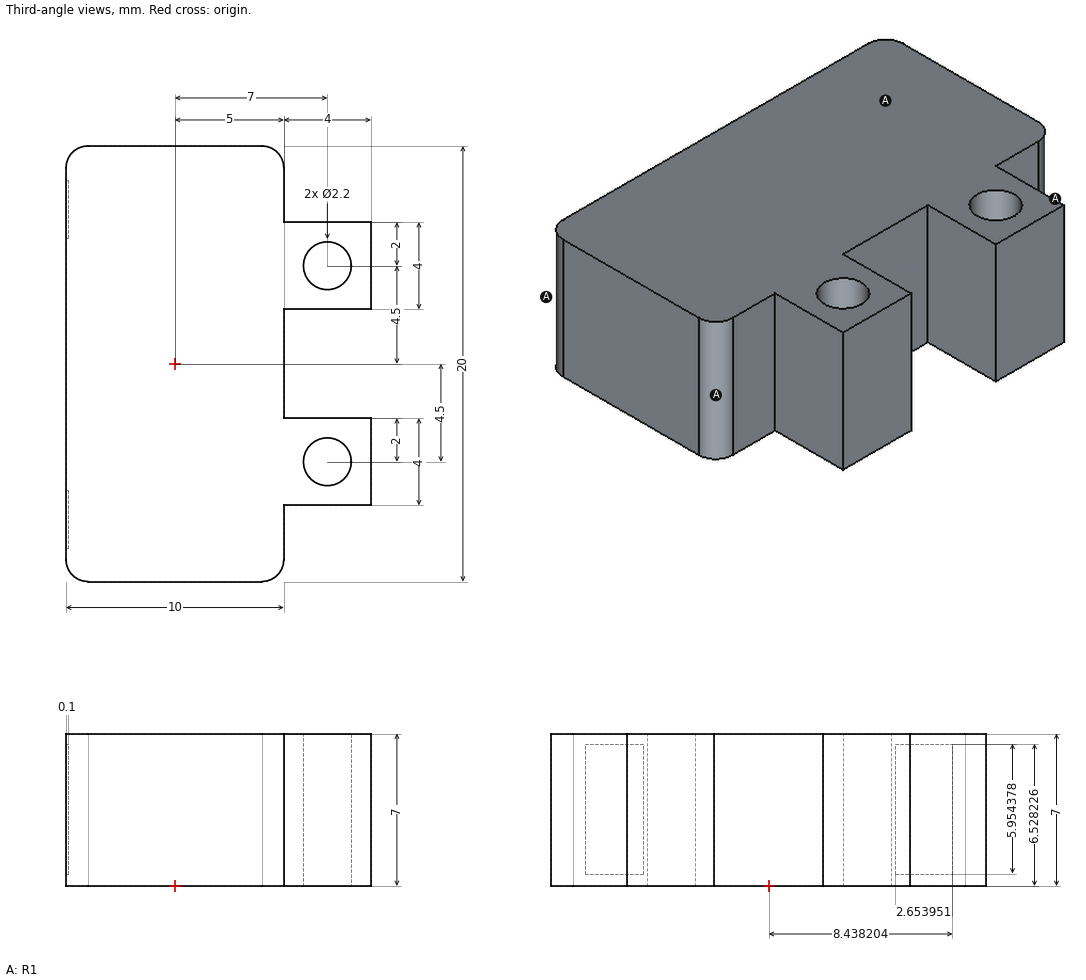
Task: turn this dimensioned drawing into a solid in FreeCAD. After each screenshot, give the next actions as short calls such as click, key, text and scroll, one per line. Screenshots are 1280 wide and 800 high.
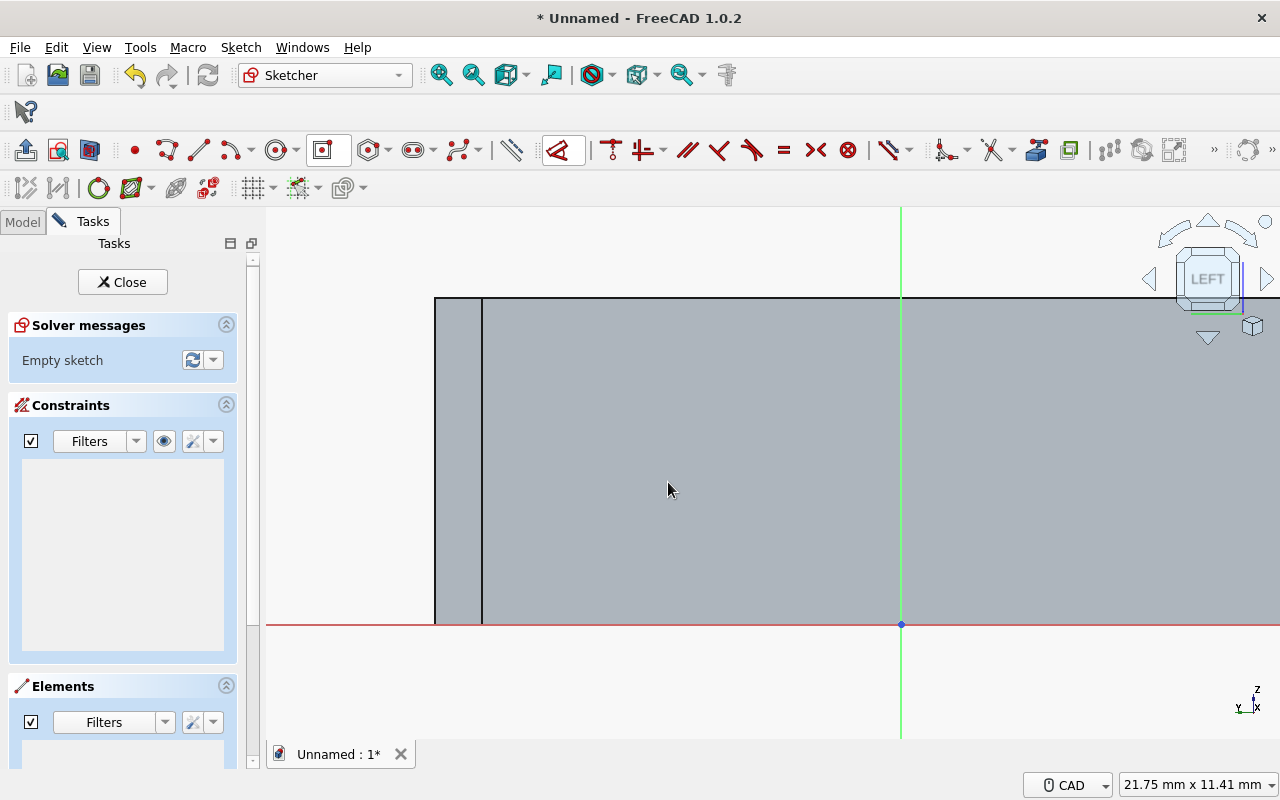
key(g)
key(r)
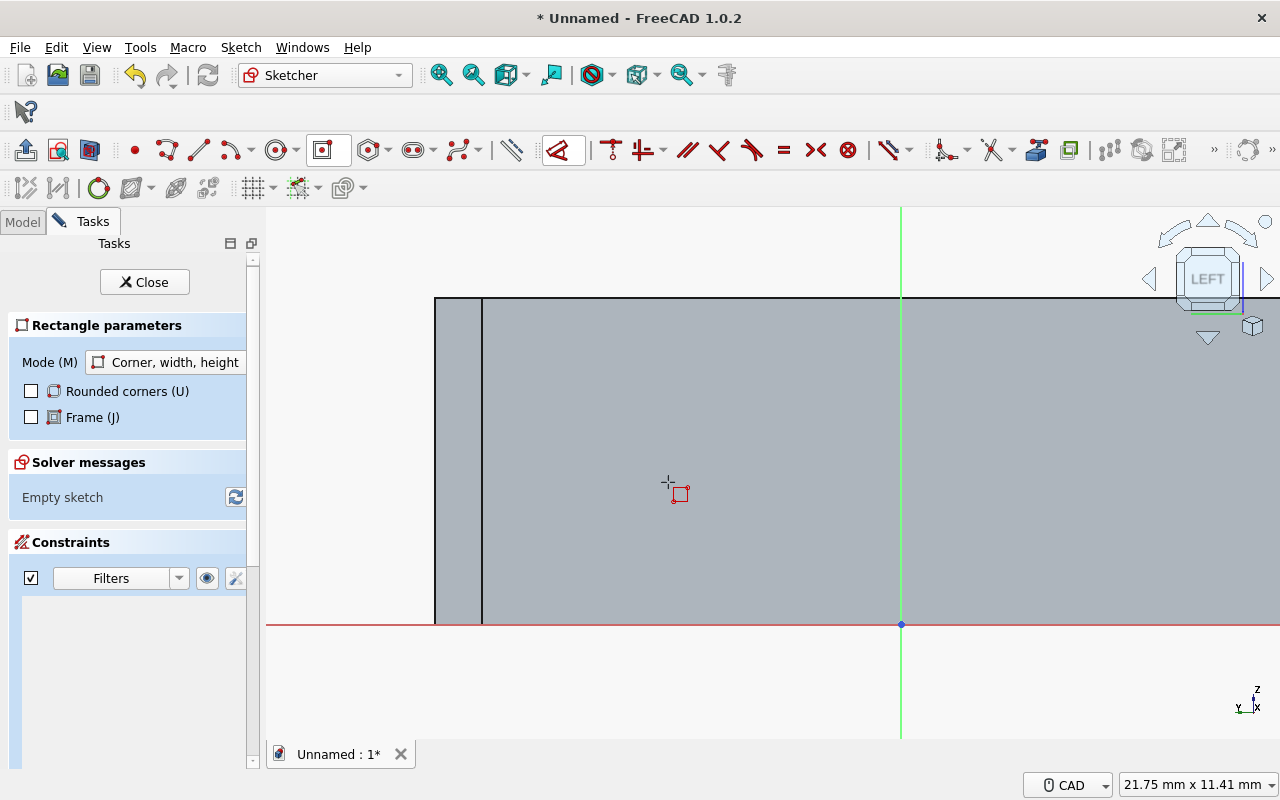
click(508, 320)
click(632, 598)
key(Escape)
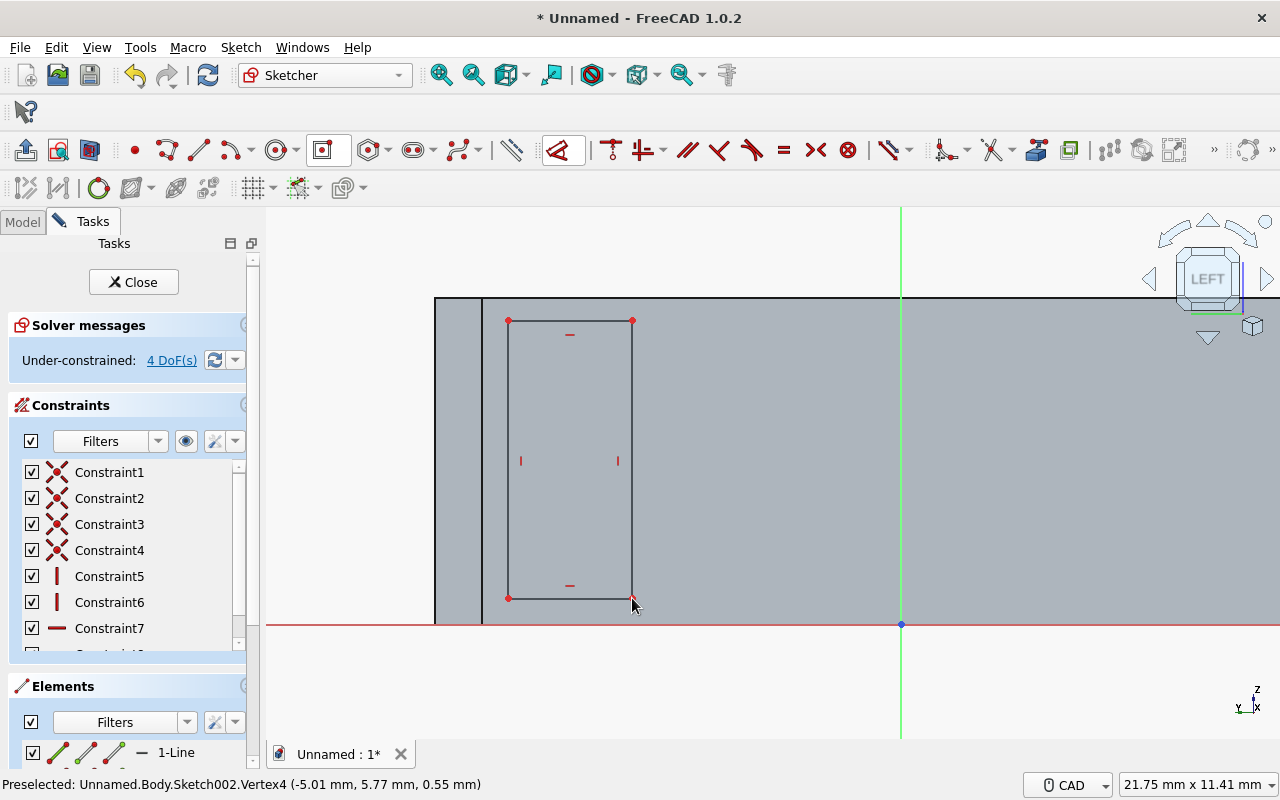
click(508, 404)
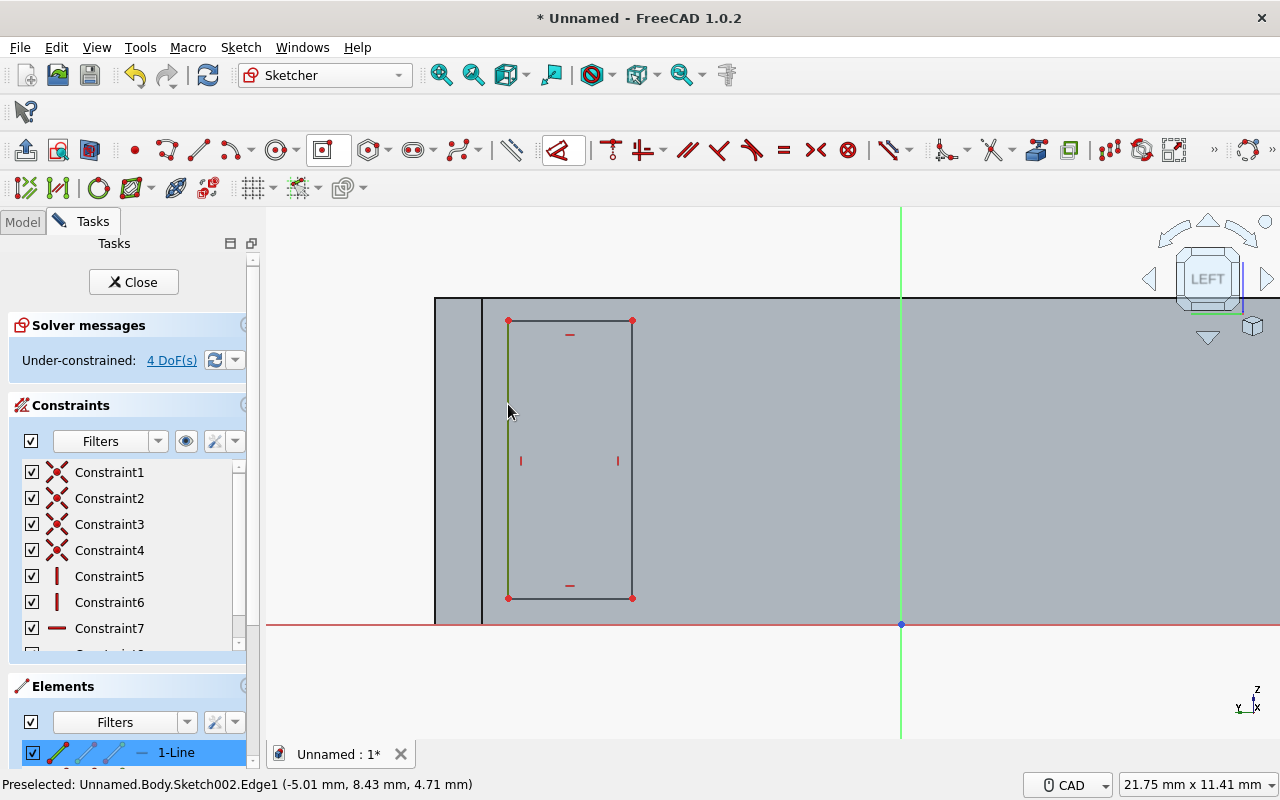
click(580, 150)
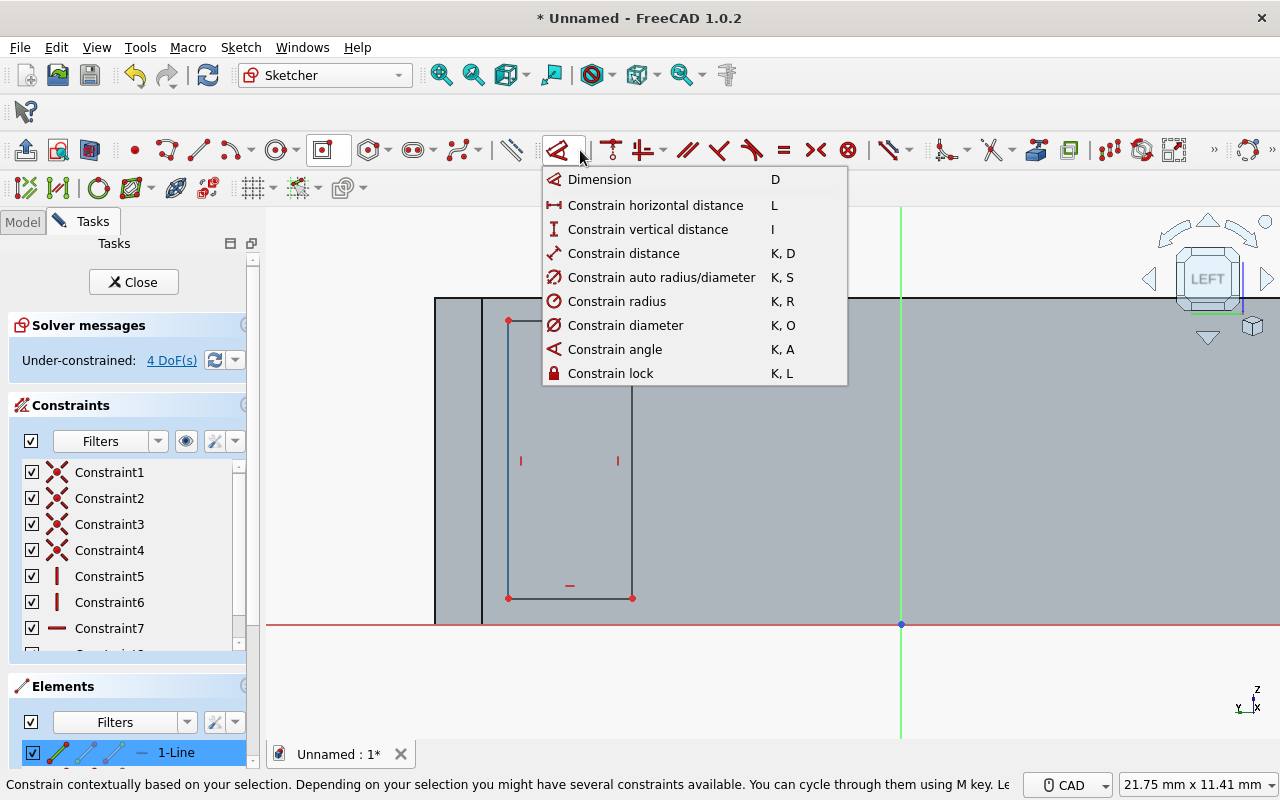
click(695, 229)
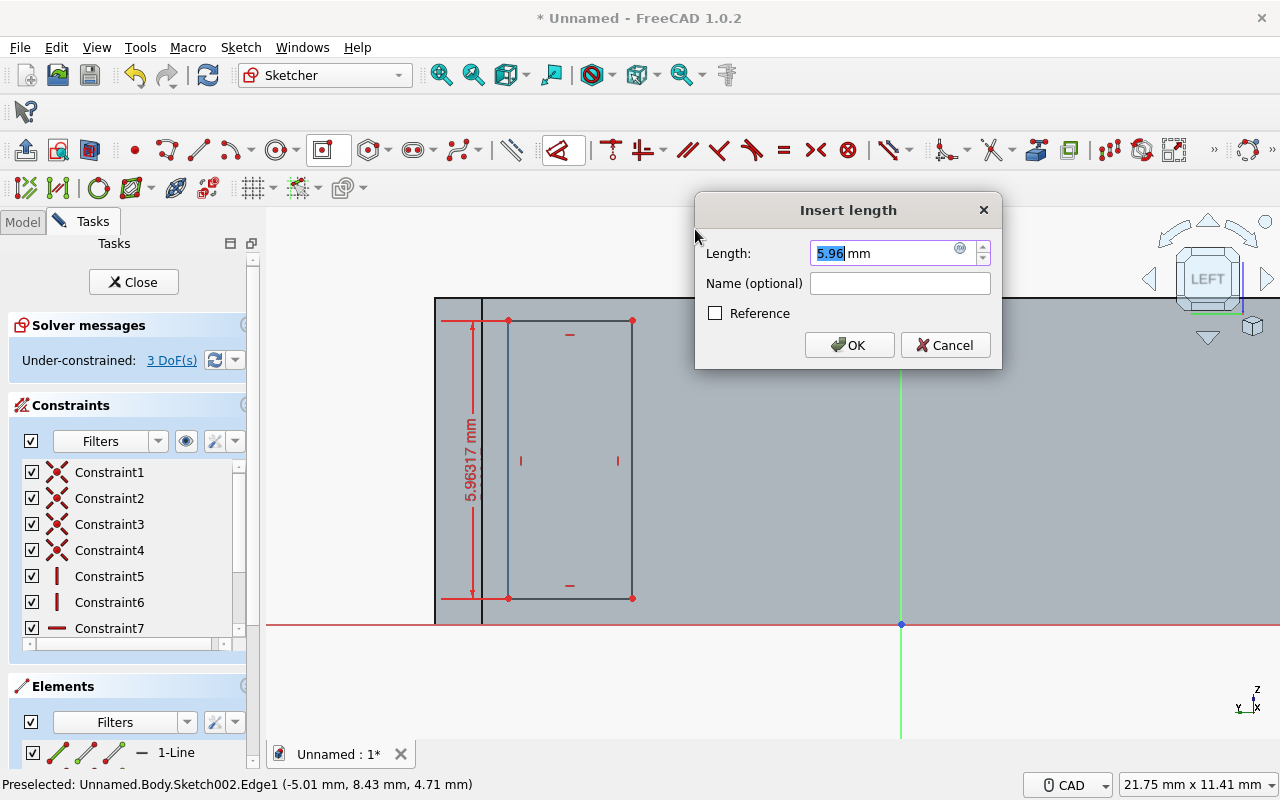
text(5.954378)
key(Return)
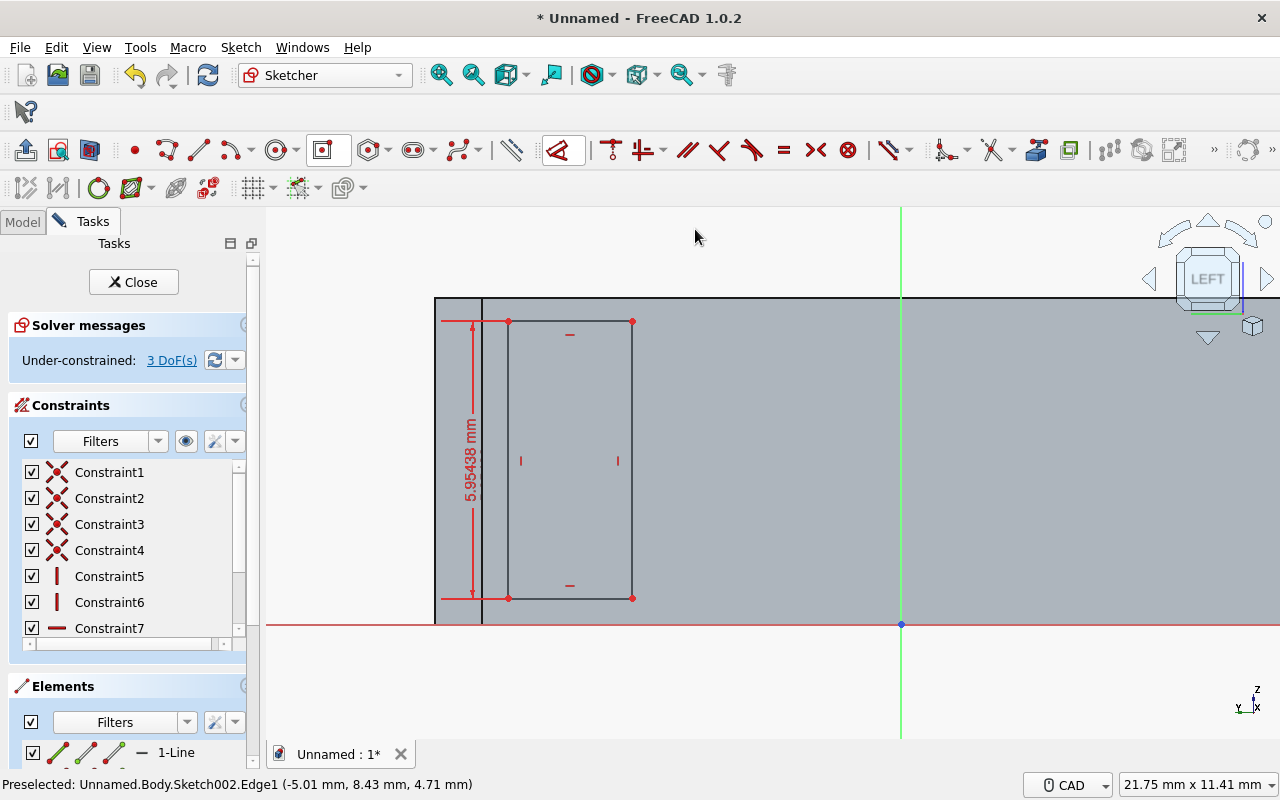
click(545, 599)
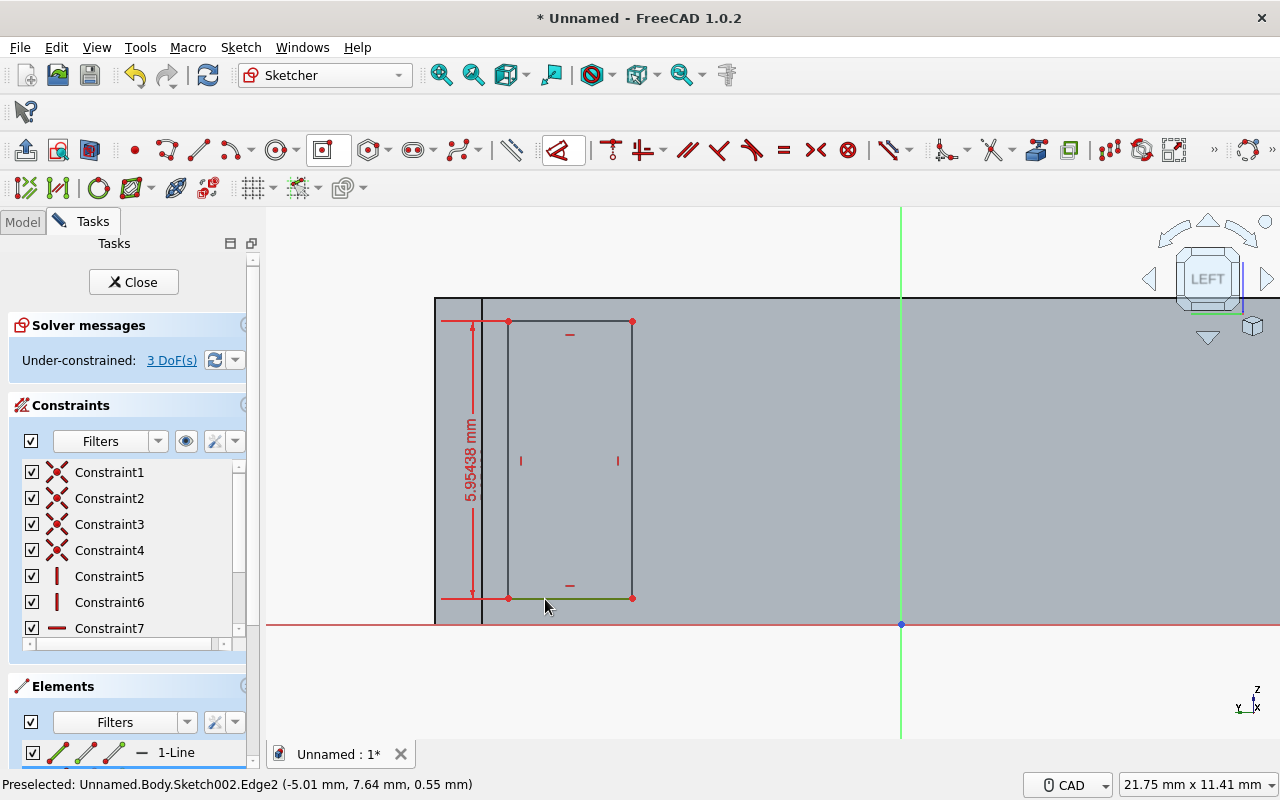
key(l)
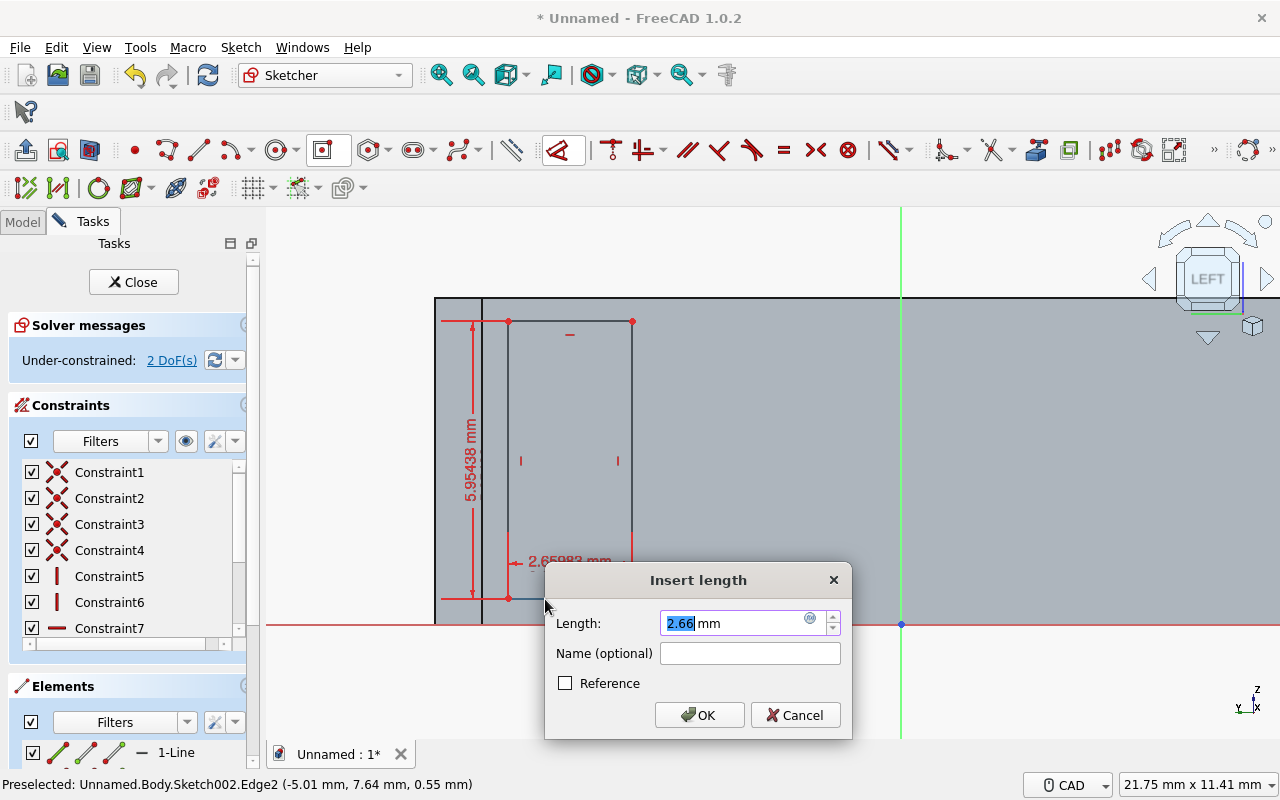
text(2.653951)
key(Return)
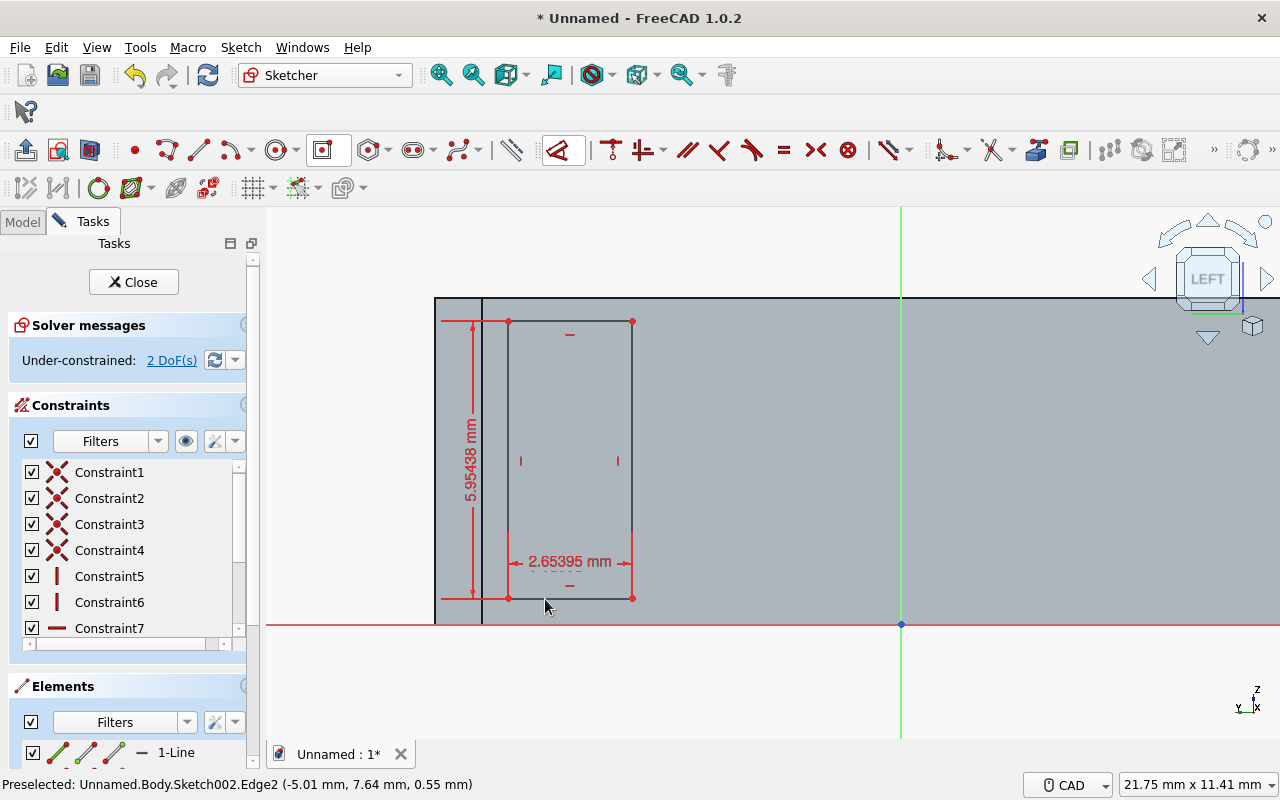
click(508, 321)